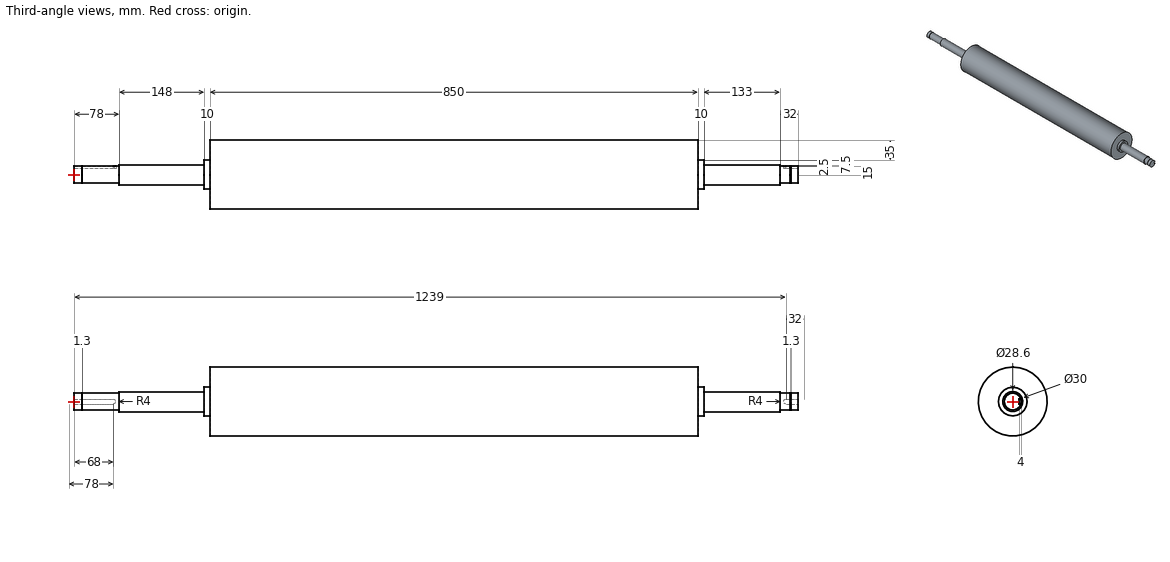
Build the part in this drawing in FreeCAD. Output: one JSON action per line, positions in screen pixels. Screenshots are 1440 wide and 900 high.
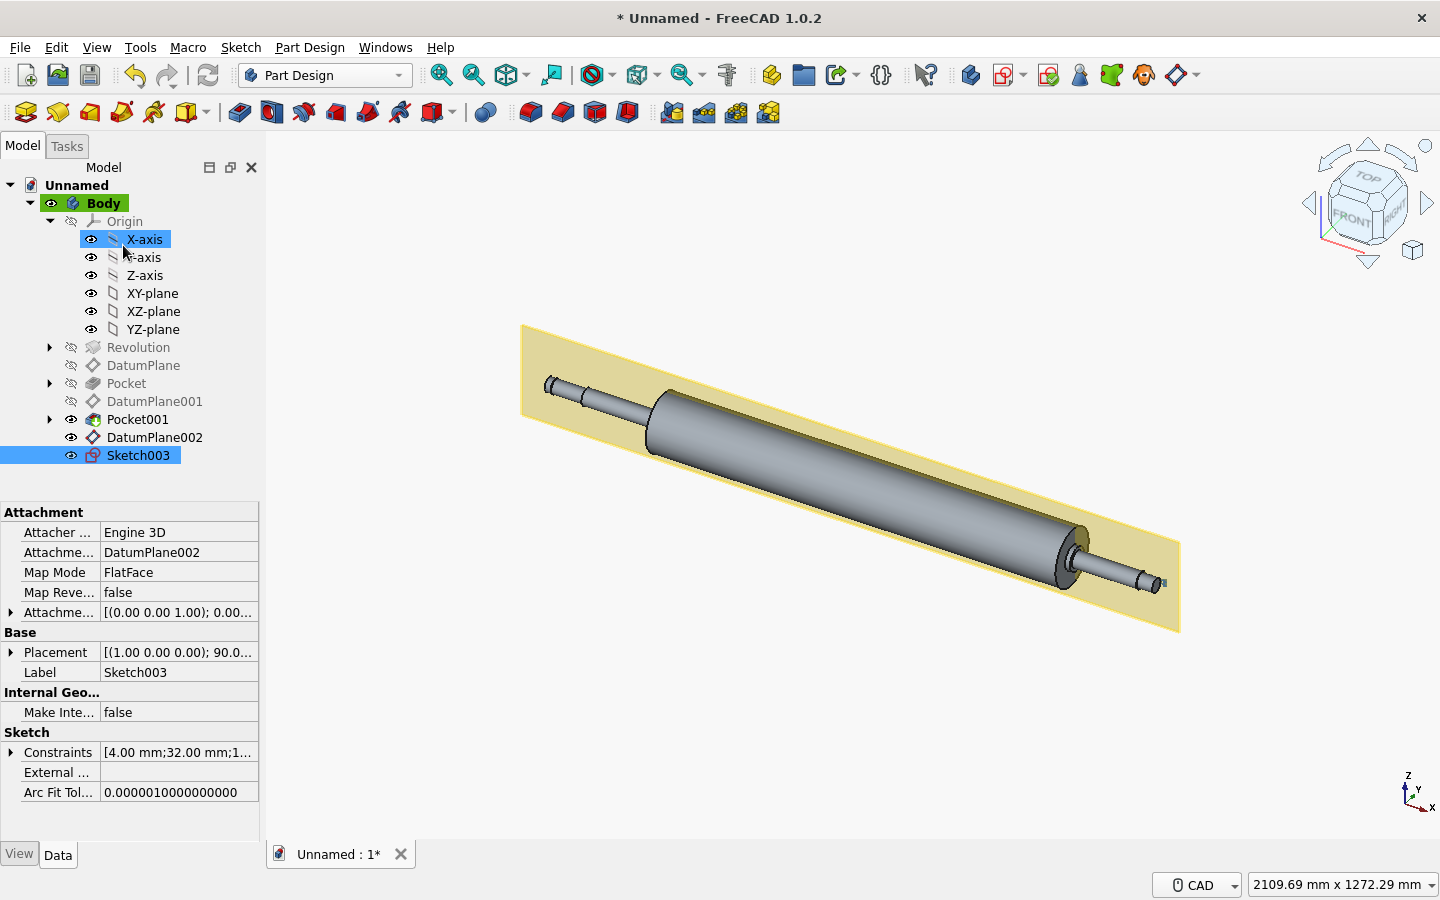
{"action": "left_click", "coordinate": [240, 112]}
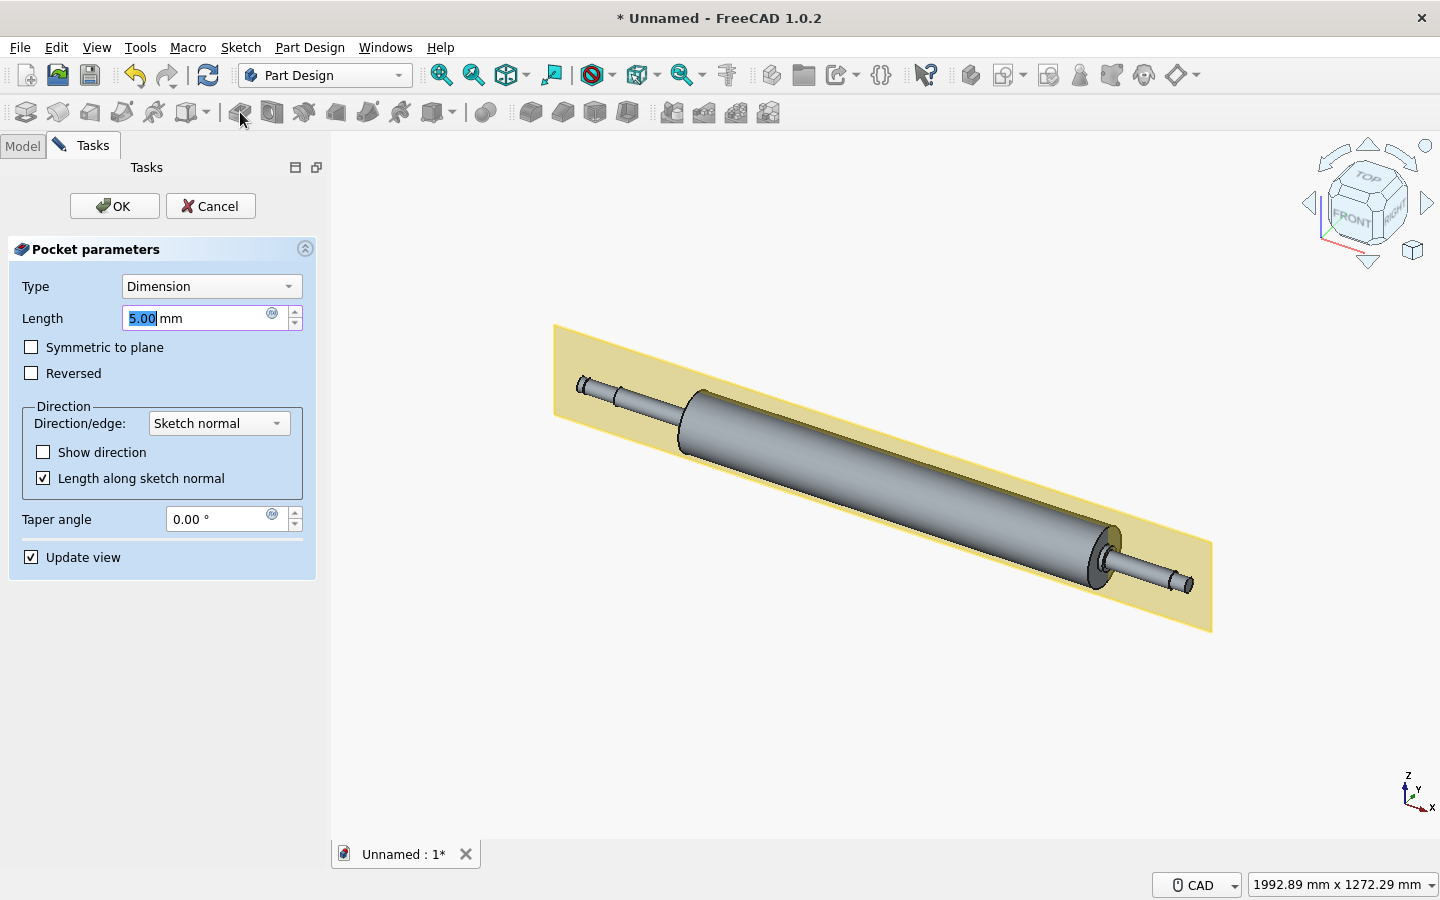
{"action": "type", "text": "4"}
{"action": "key", "text": "Tab"}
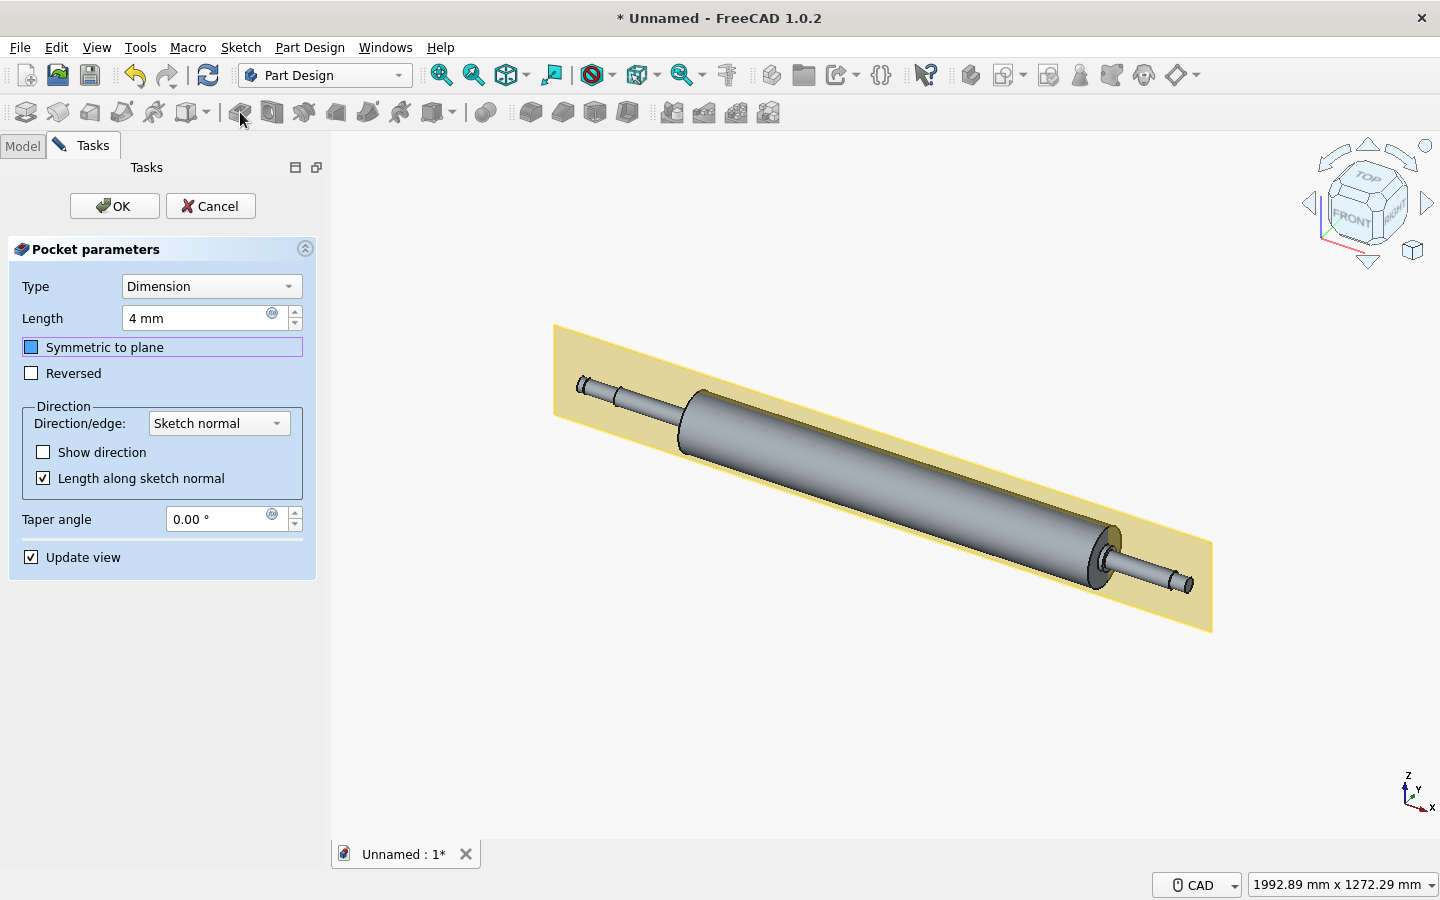
{"action": "left_click", "coordinate": [30, 373]}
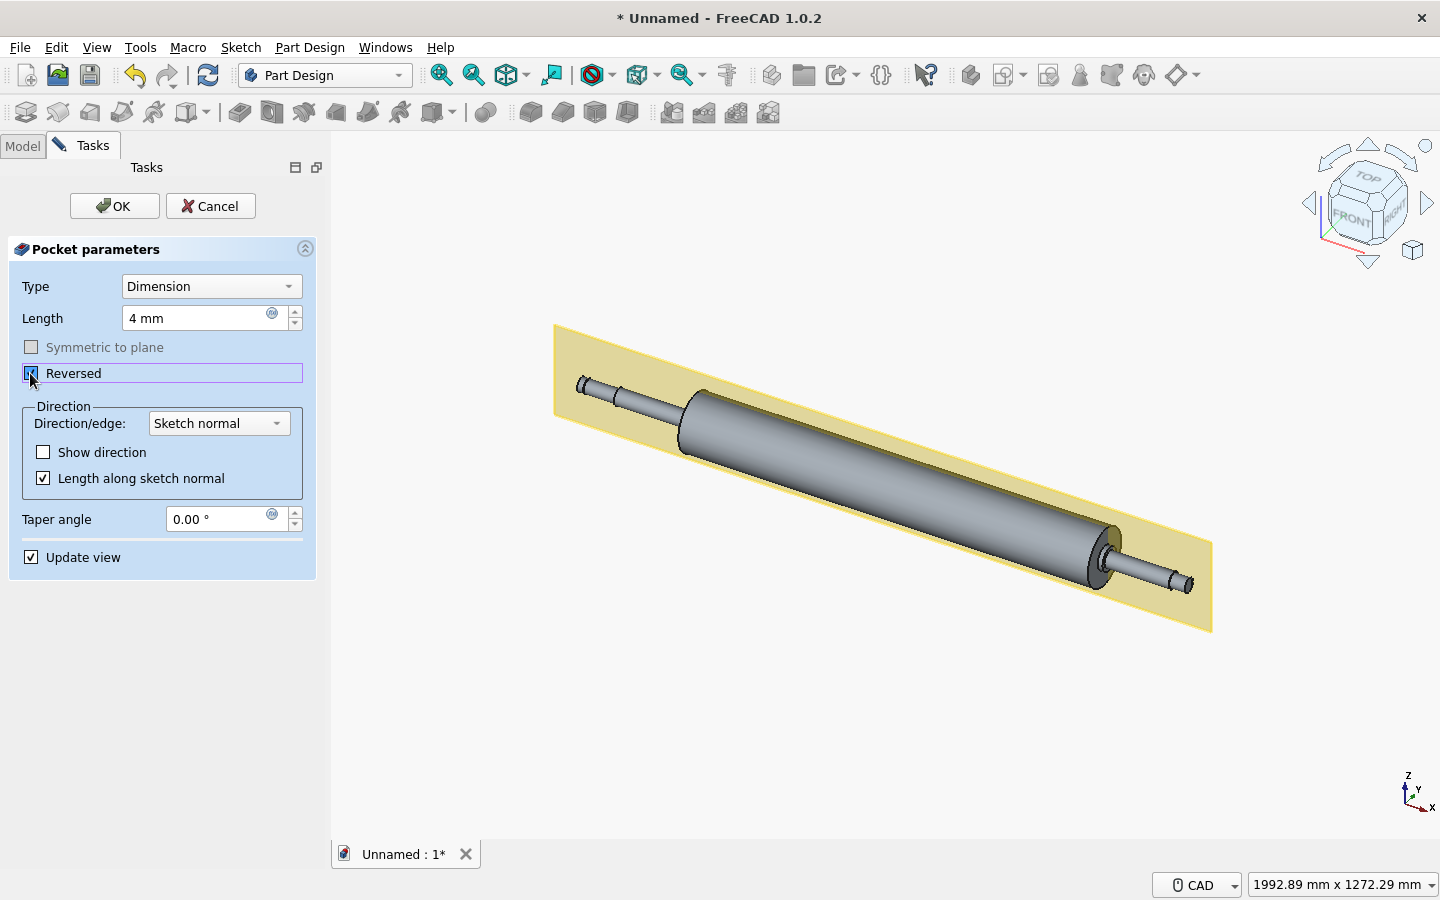
{"action": "left_click", "coordinate": [115, 206]}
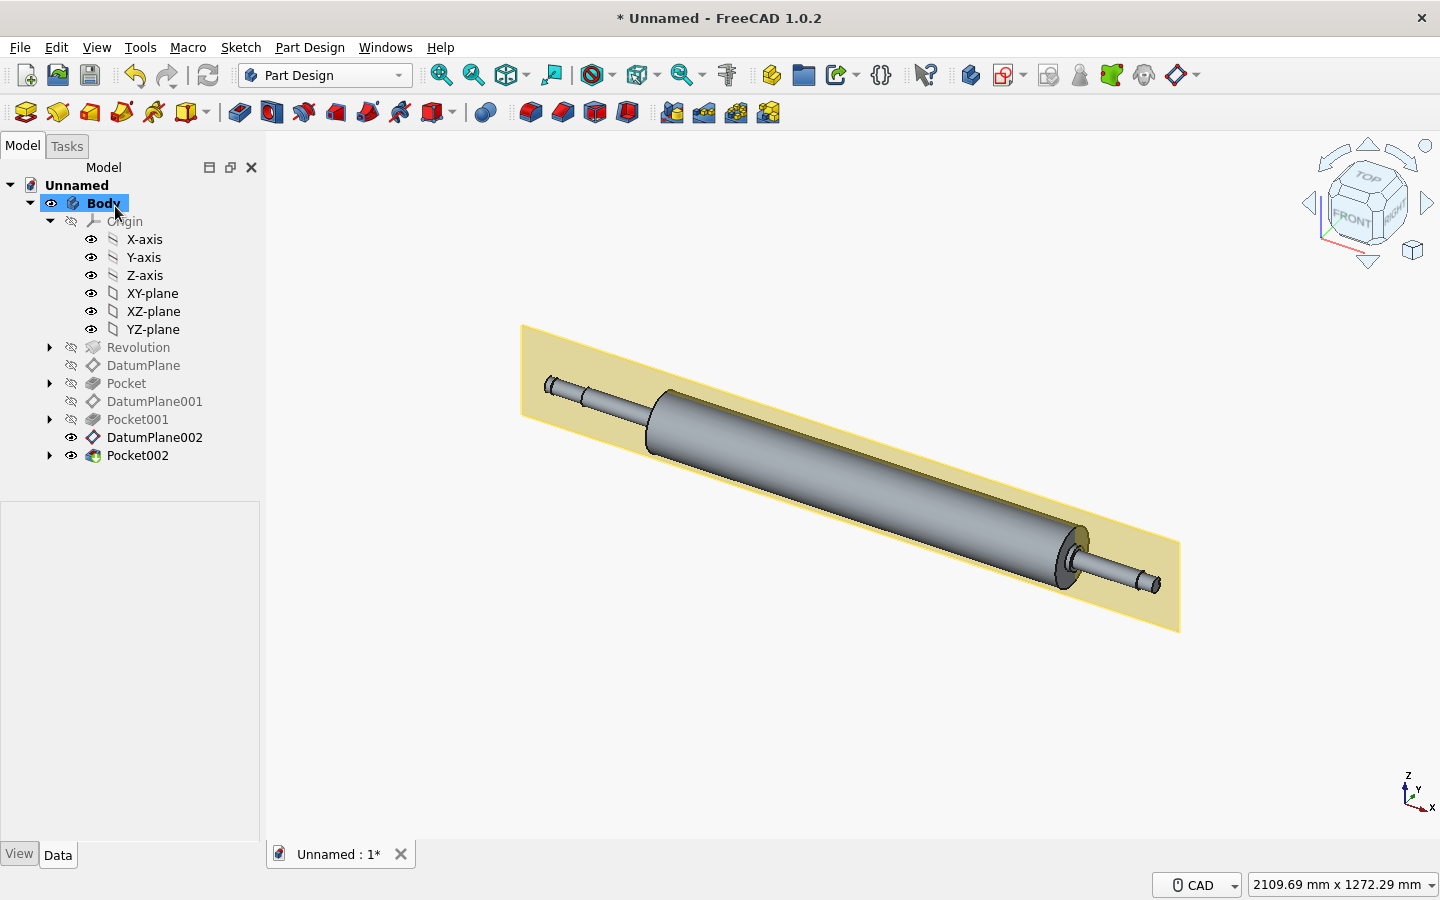
{"action": "left_click", "coordinate": [116, 437]}
{"action": "key", "text": "space"}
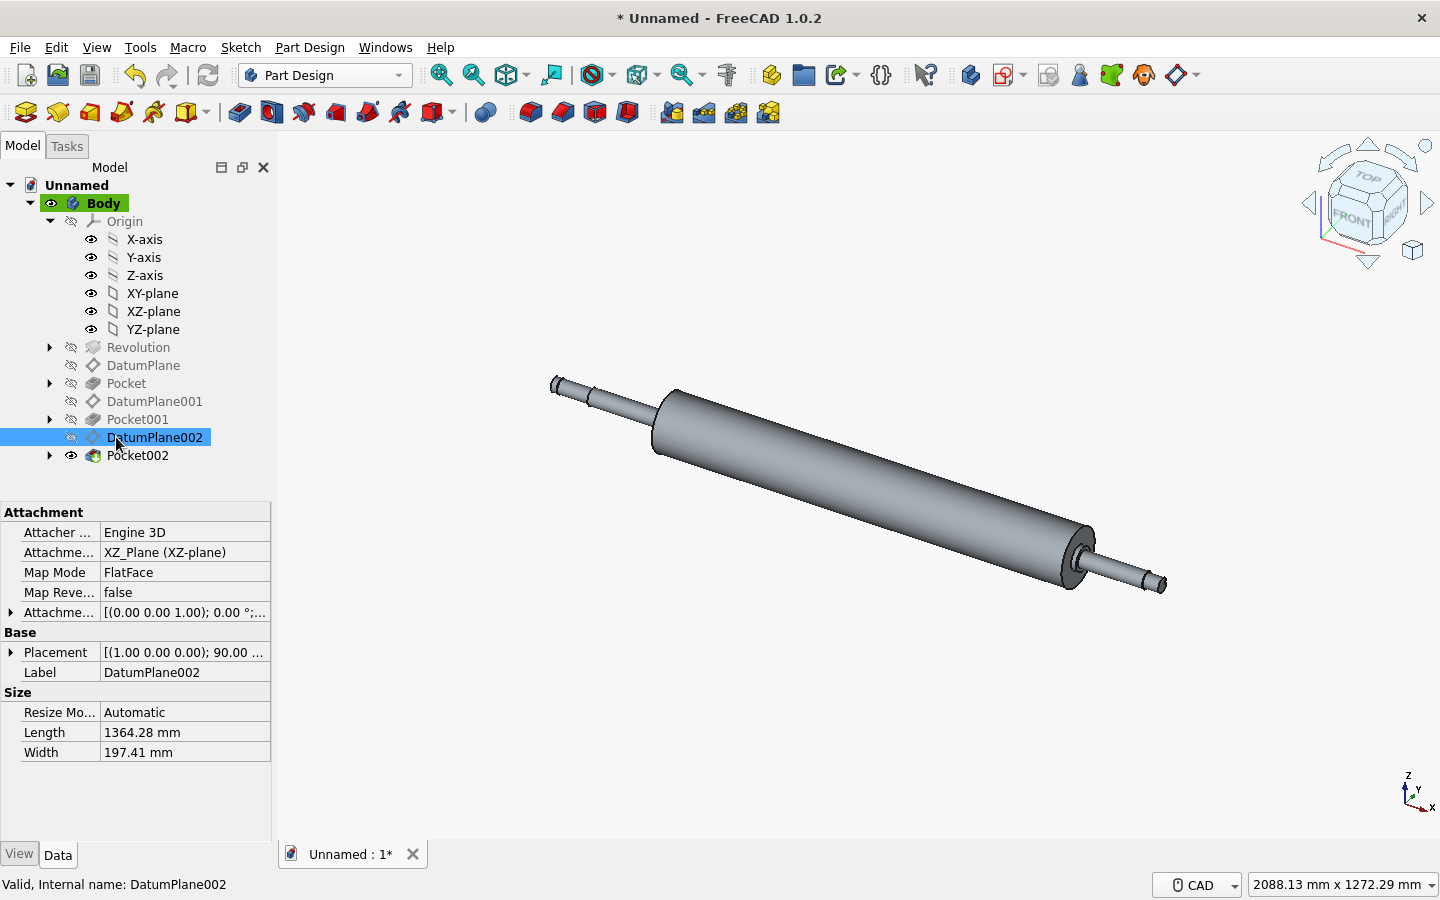
{"action": "left_click", "coordinate": [136, 329]}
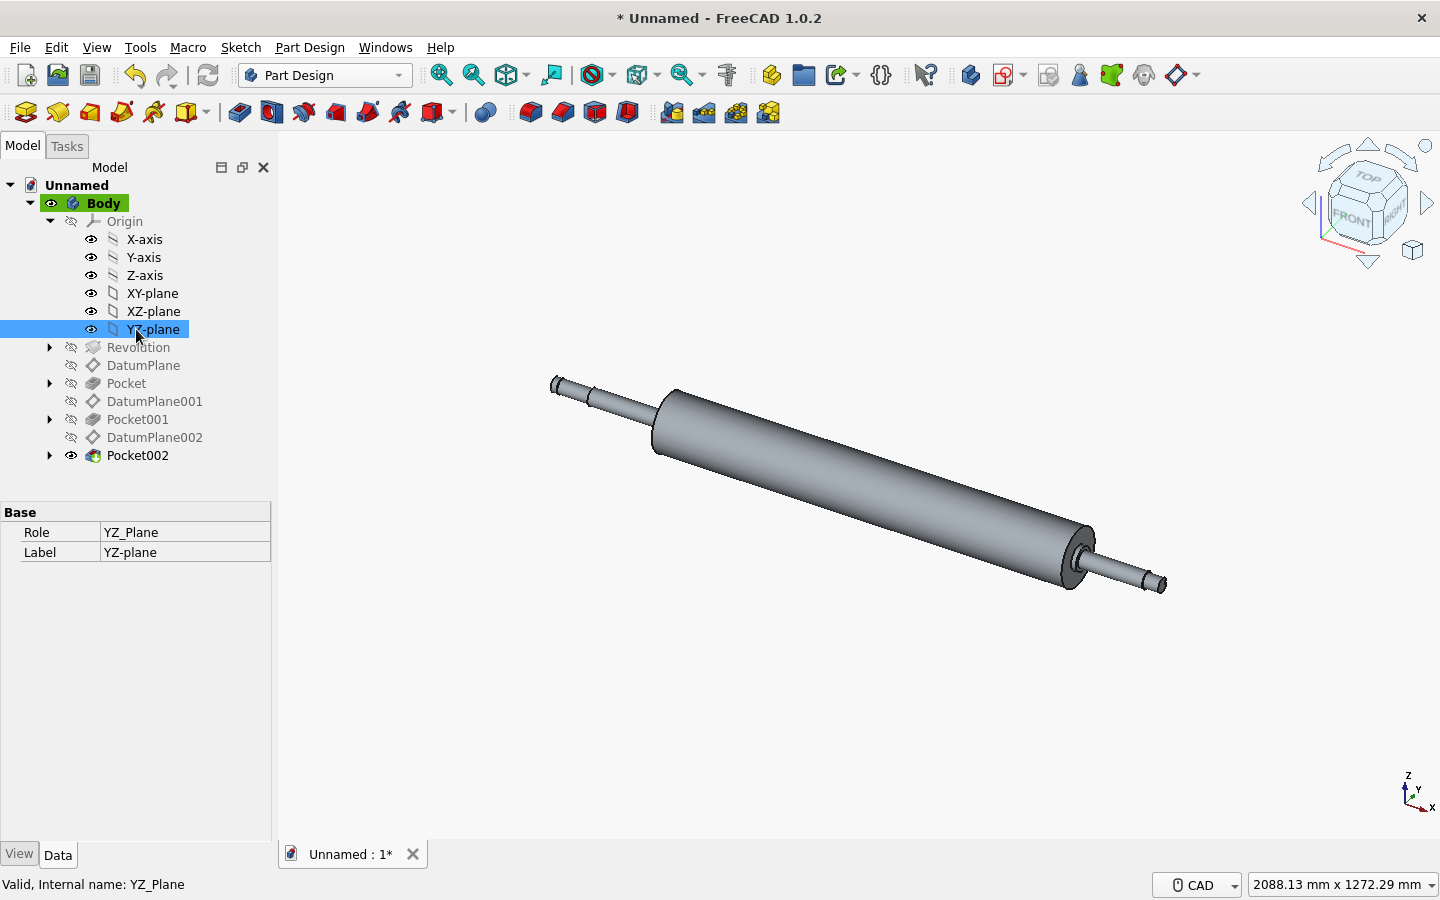
{"action": "left_click", "coordinate": [1176, 76]}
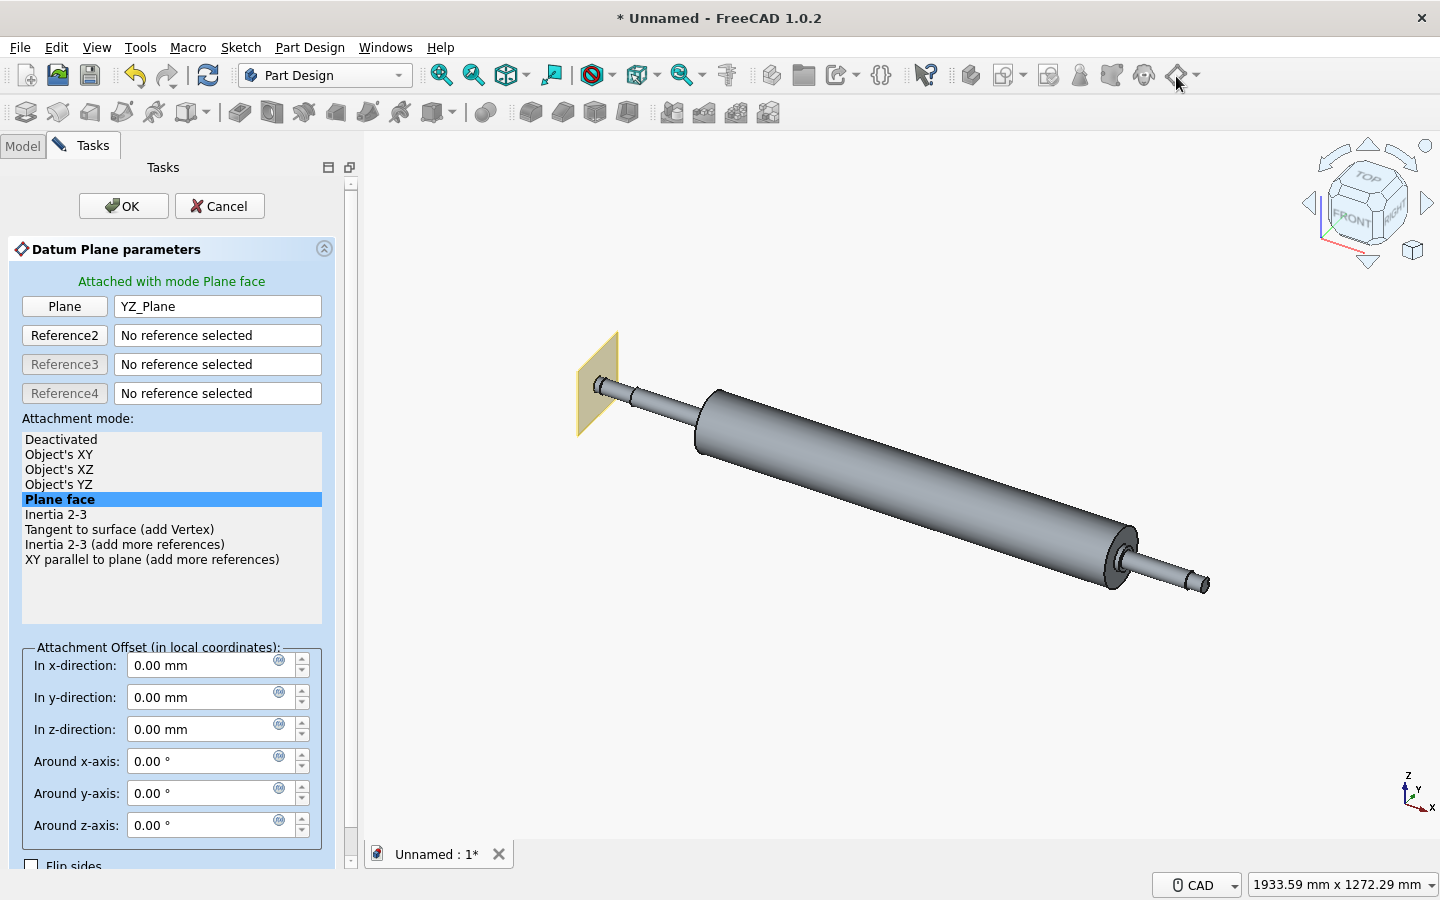
{"action": "triple_click", "coordinate": [210, 729]}